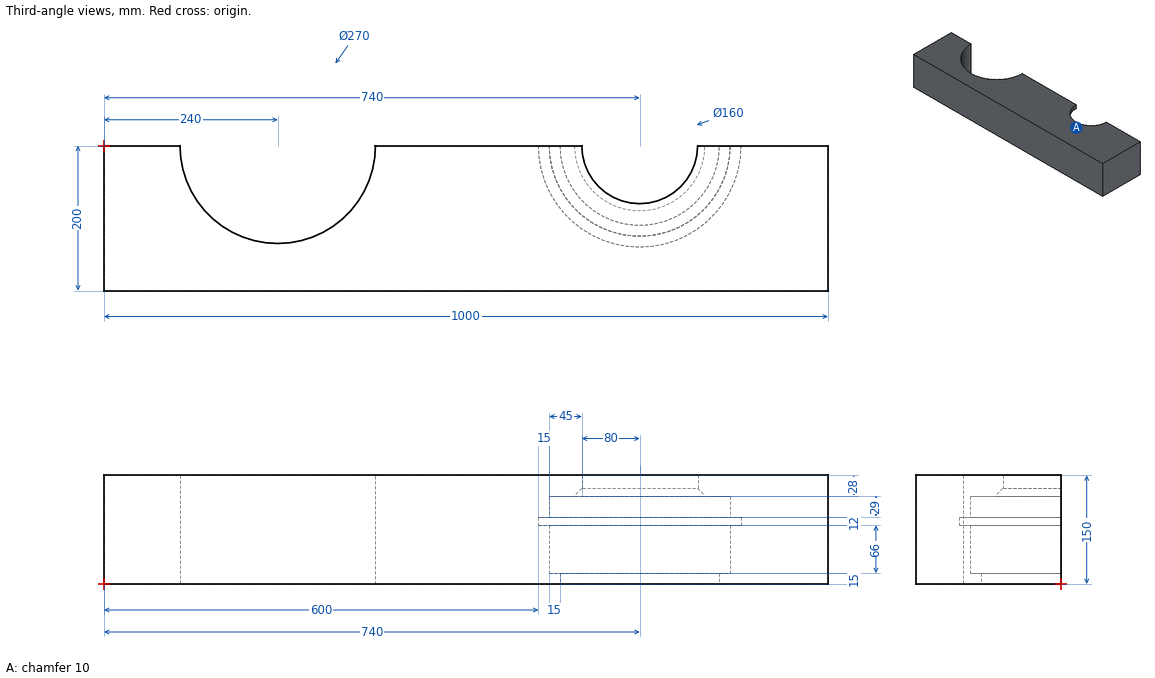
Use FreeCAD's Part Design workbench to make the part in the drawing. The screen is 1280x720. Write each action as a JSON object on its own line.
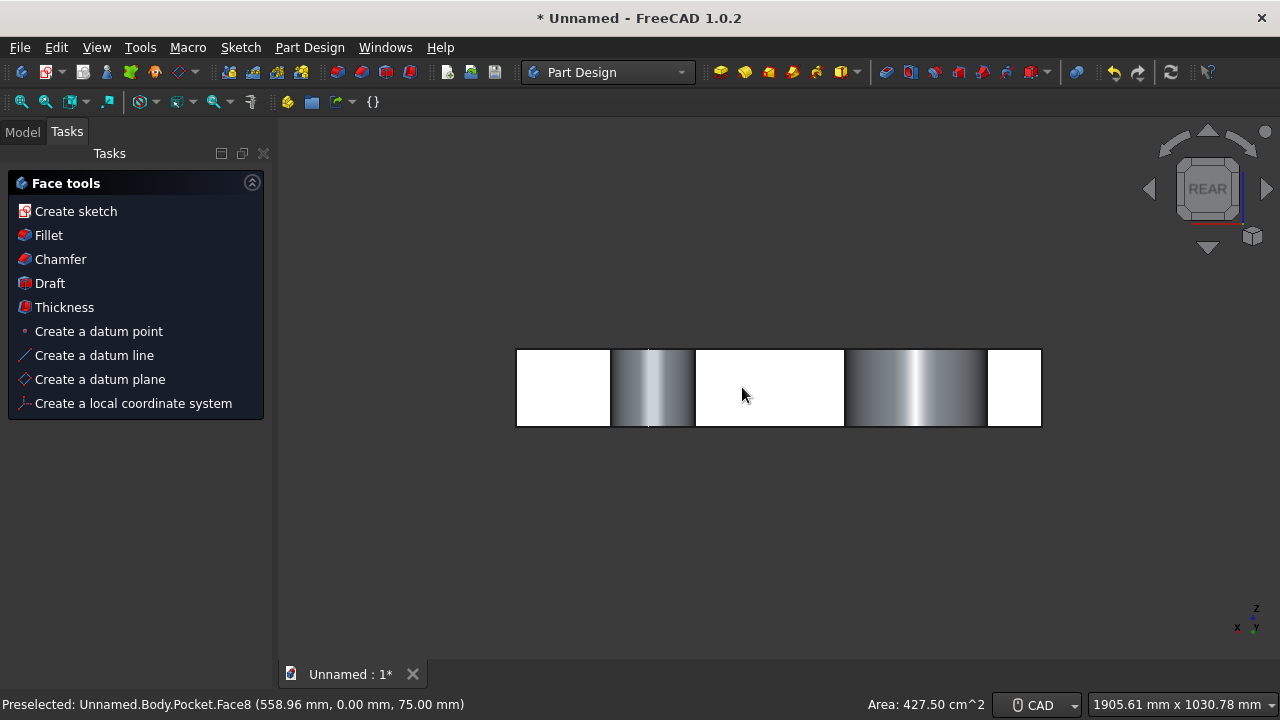
{"action": "left_click", "coordinate": [46, 72]}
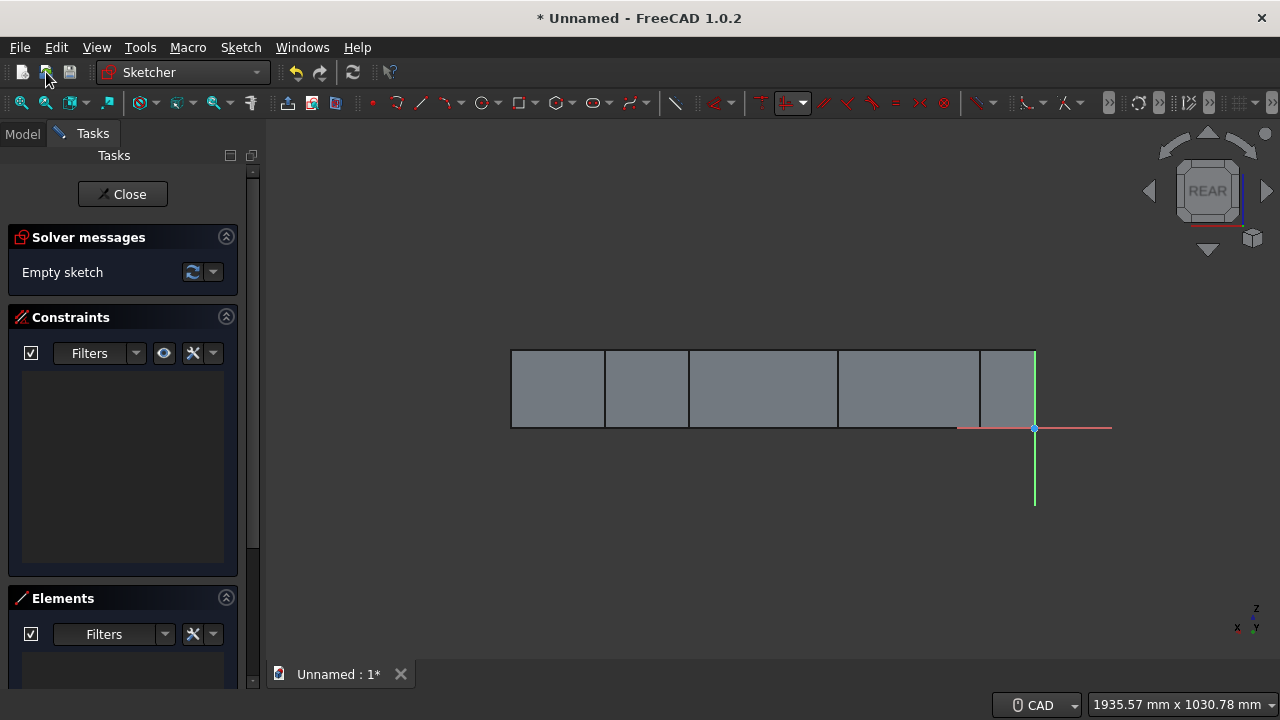
{"action": "scroll", "coordinate": [675, 367], "scroll_direction": "up", "scroll_amount": 6}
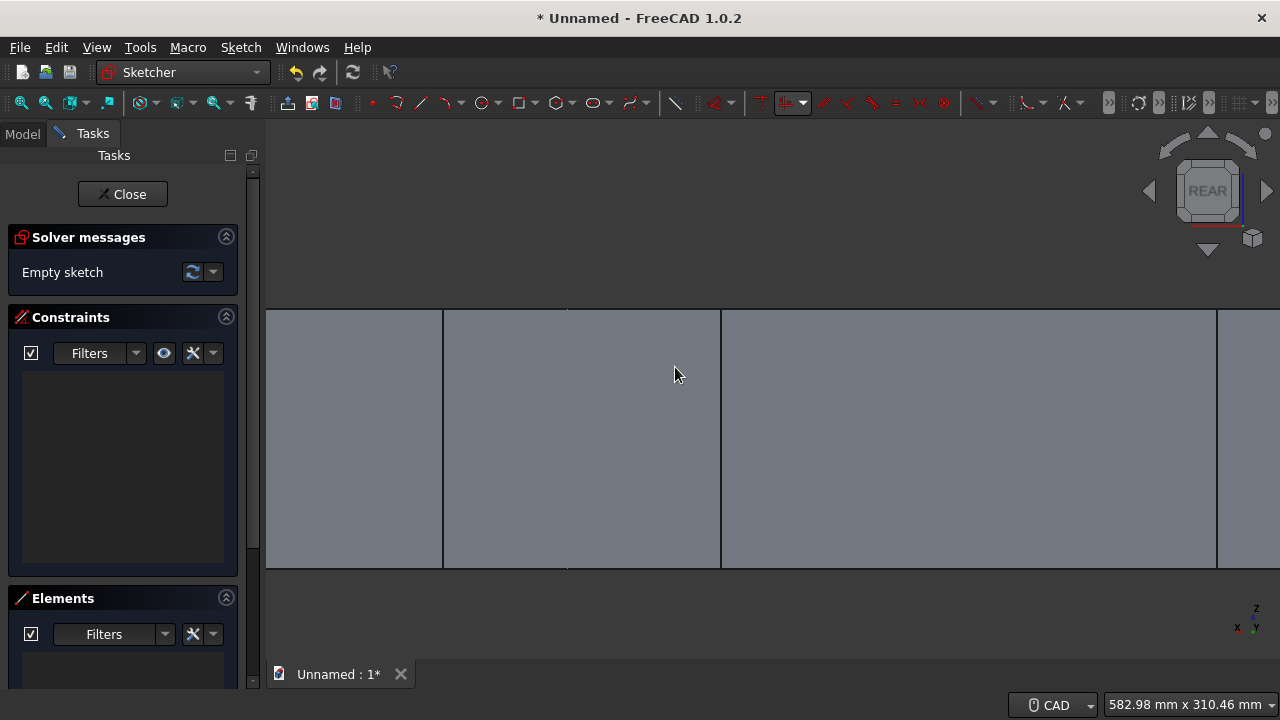
{"action": "left_click", "coordinate": [398, 104]}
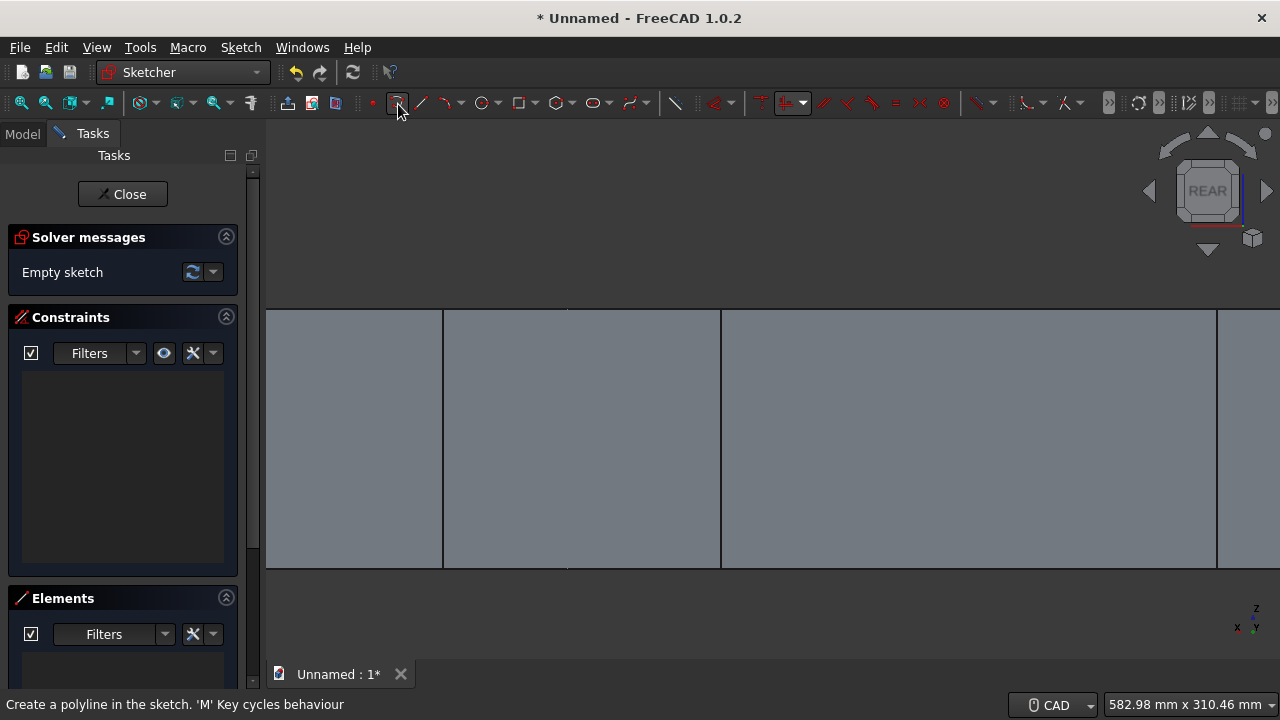
{"action": "left_click", "coordinate": [826, 429]}
{"action": "left_click", "coordinate": [826, 408]}
{"action": "left_click", "coordinate": [799, 408]}
{"action": "left_click", "coordinate": [799, 357]}
{"action": "left_click", "coordinate": [721, 357]}
{"action": "left_click", "coordinate": [721, 309]}
{"action": "left_click", "coordinate": [582, 309]}
{"action": "left_click", "coordinate": [582, 569]}
{"action": "left_click", "coordinate": [773, 560]}
{"action": "left_click", "coordinate": [773, 543]}
{"action": "left_click", "coordinate": [799, 543]}
{"action": "left_click", "coordinate": [799, 429]}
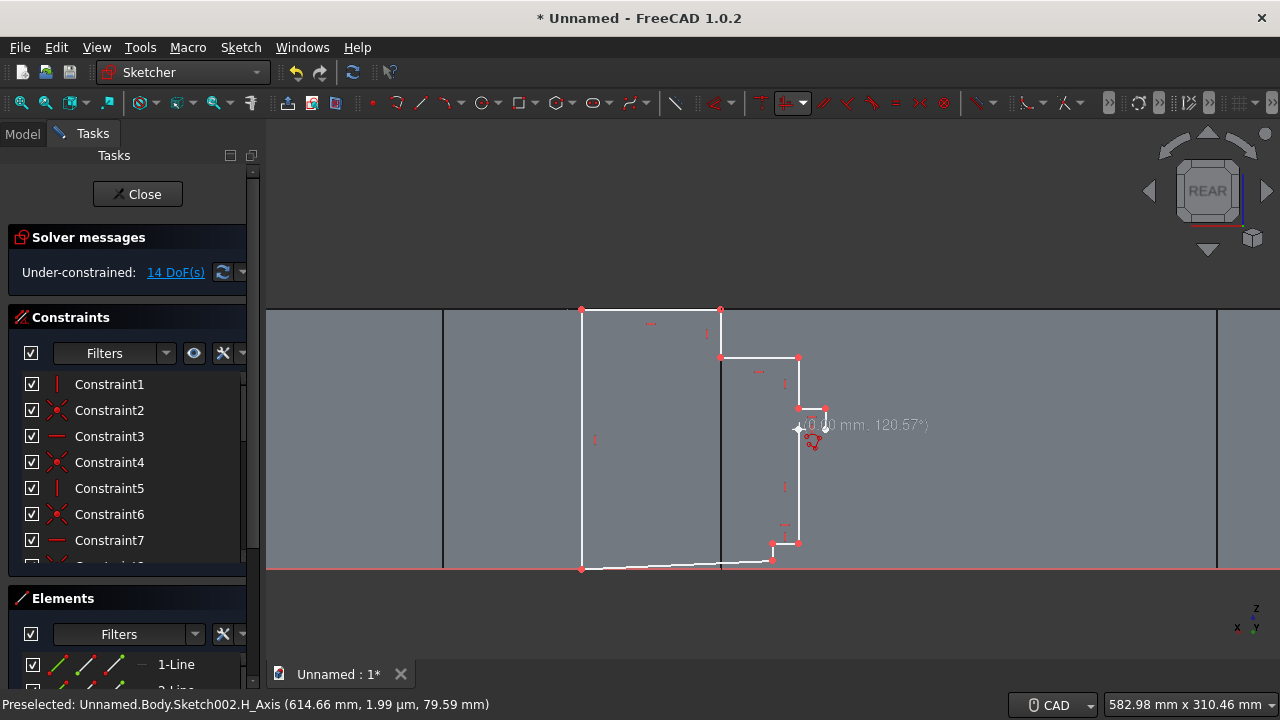
{"action": "scroll", "coordinate": [826, 429], "scroll_direction": "up", "scroll_amount": 3}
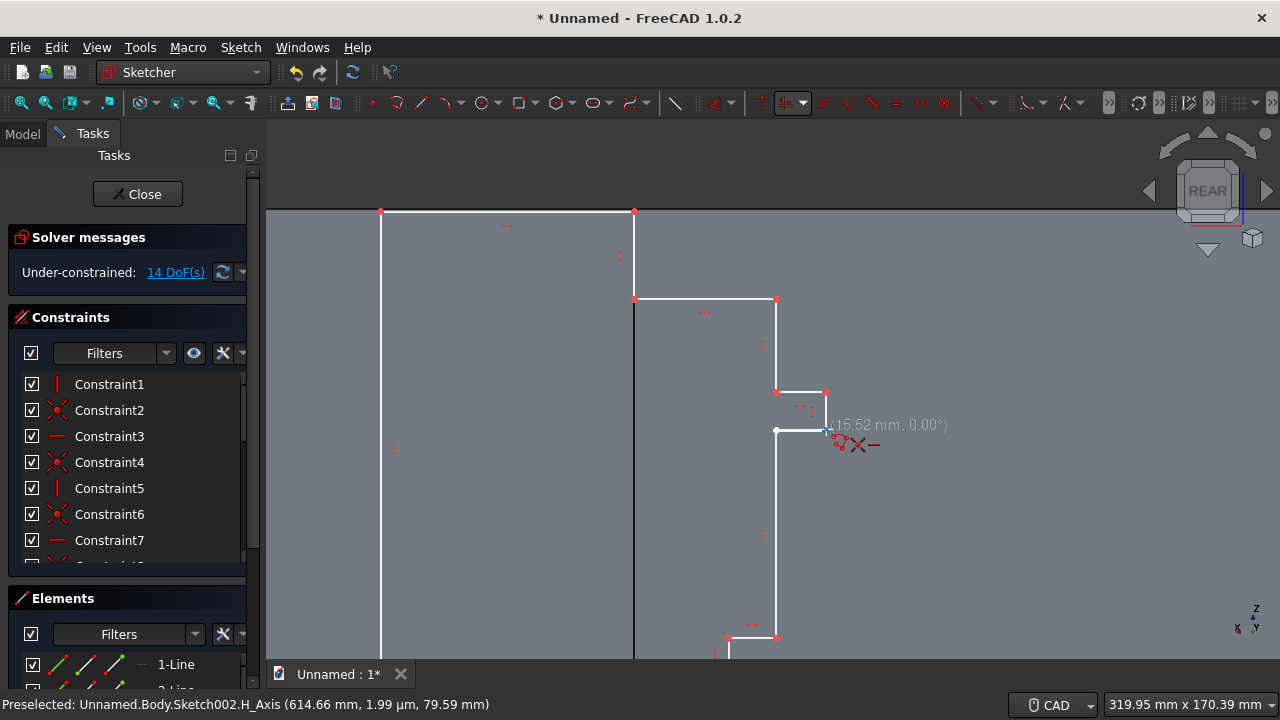
{"action": "left_click", "coordinate": [826, 430]}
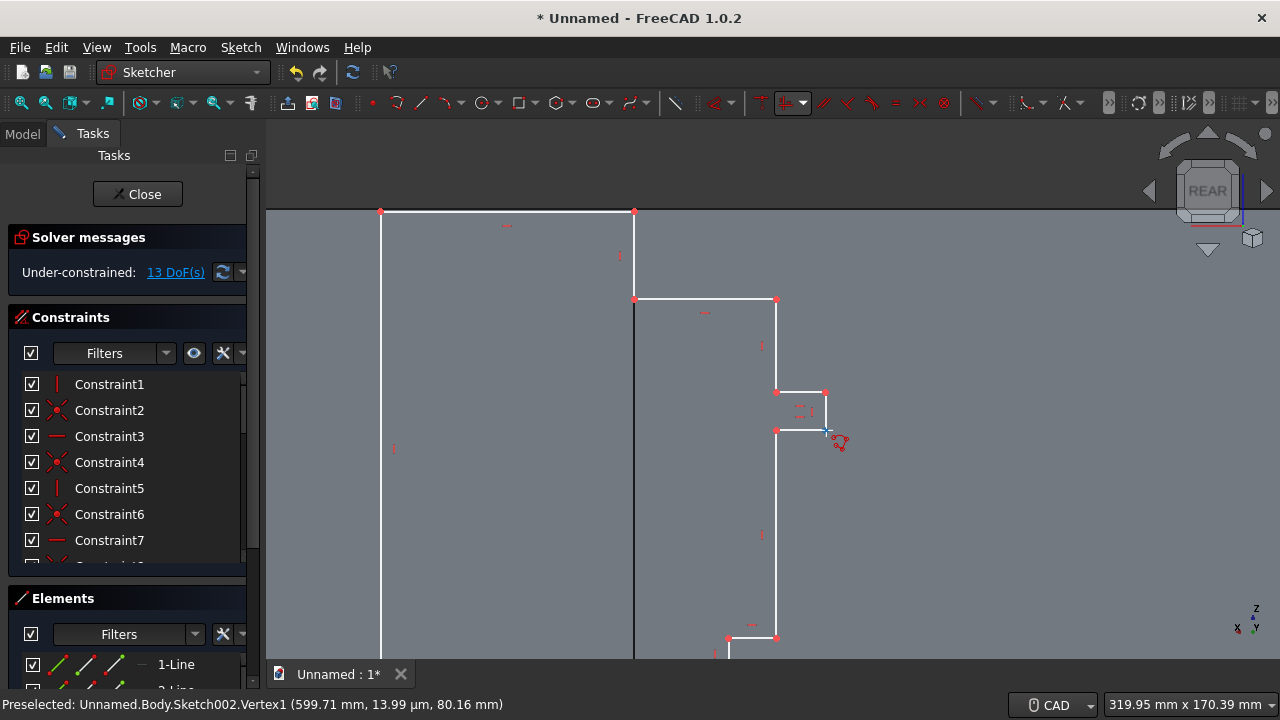
{"action": "left_click", "coordinate": [422, 104]}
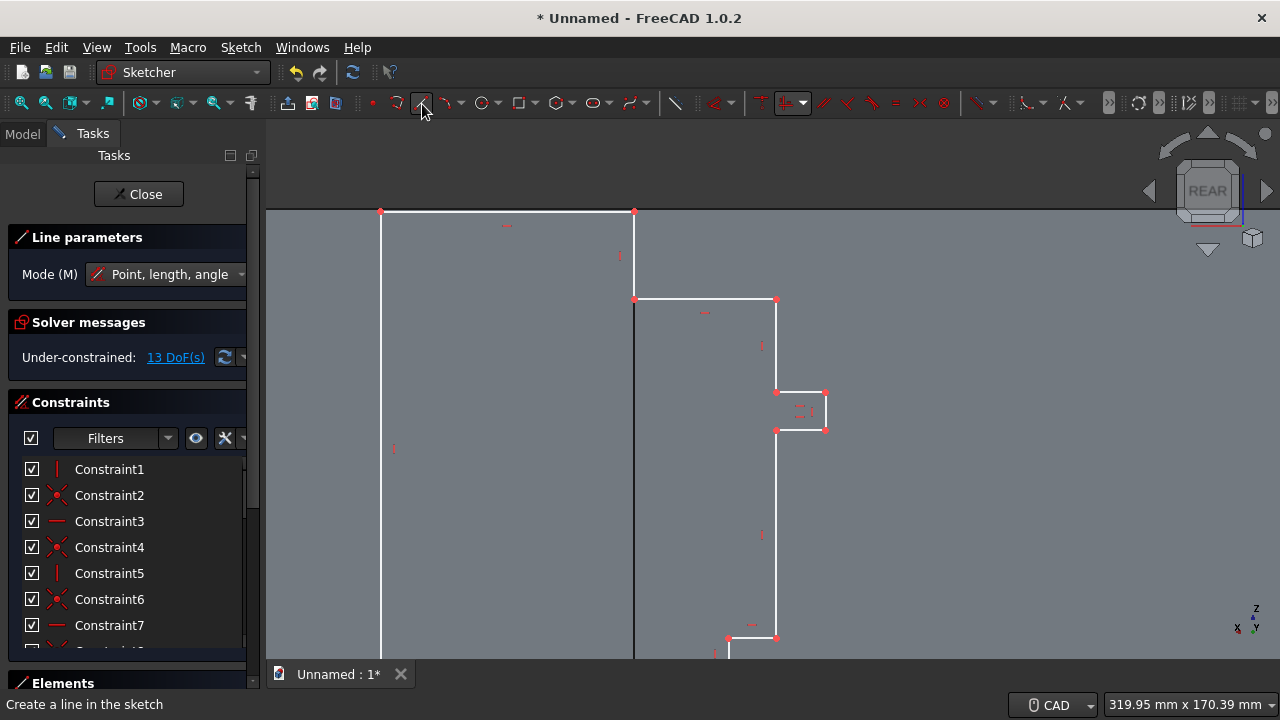
{"action": "left_click", "coordinate": [381, 161]}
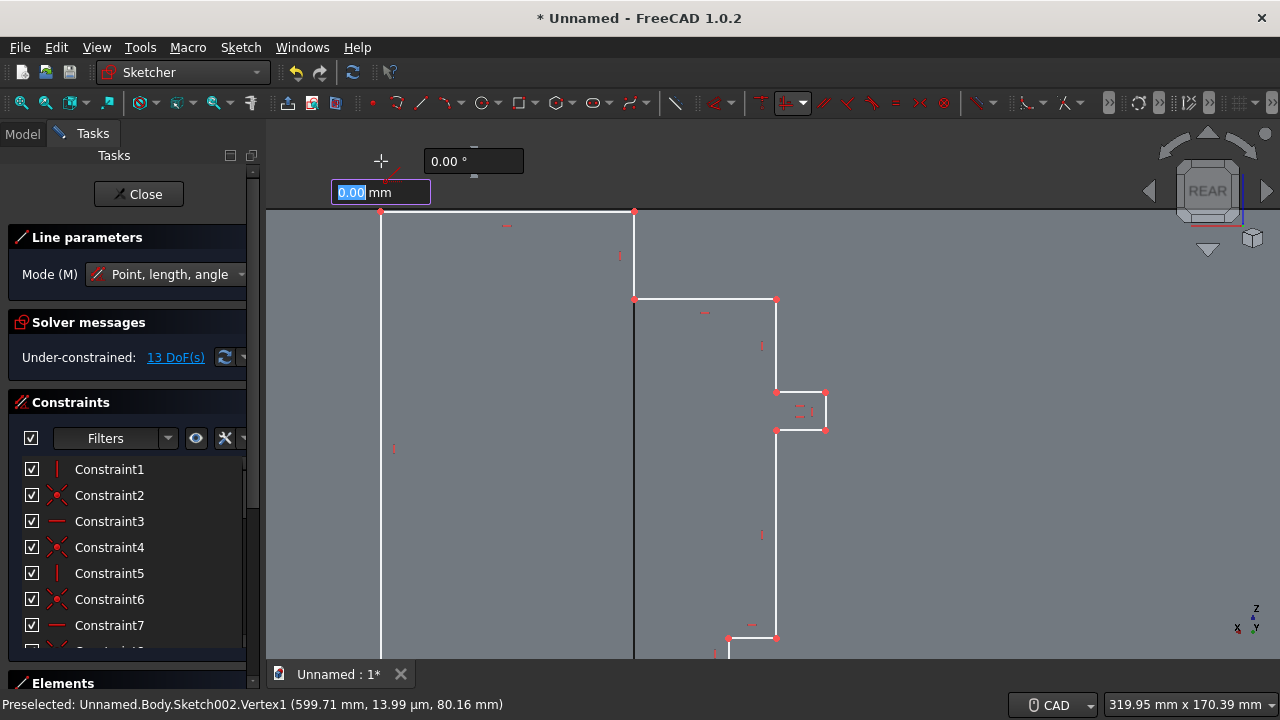
{"action": "scroll", "coordinate": [828, 434], "scroll_direction": "down", "scroll_amount": 3}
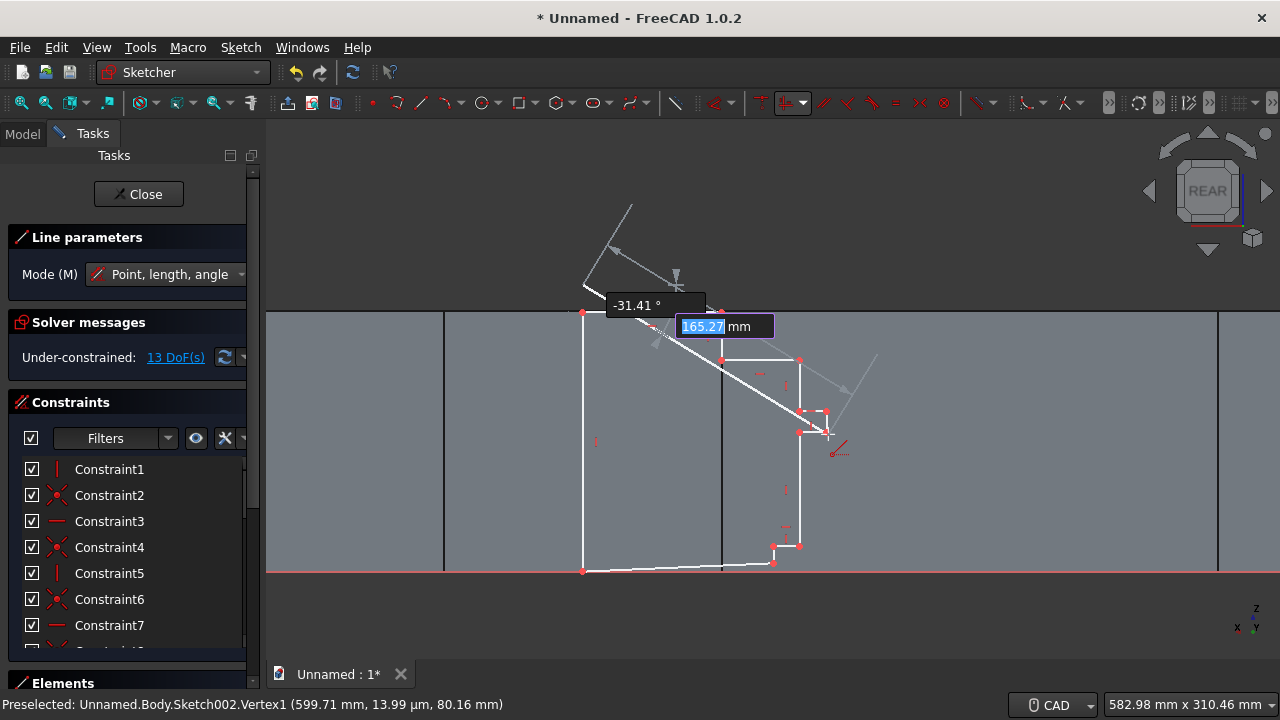
{"action": "left_click", "coordinate": [583, 206]}
{"action": "key", "text": "Escape"}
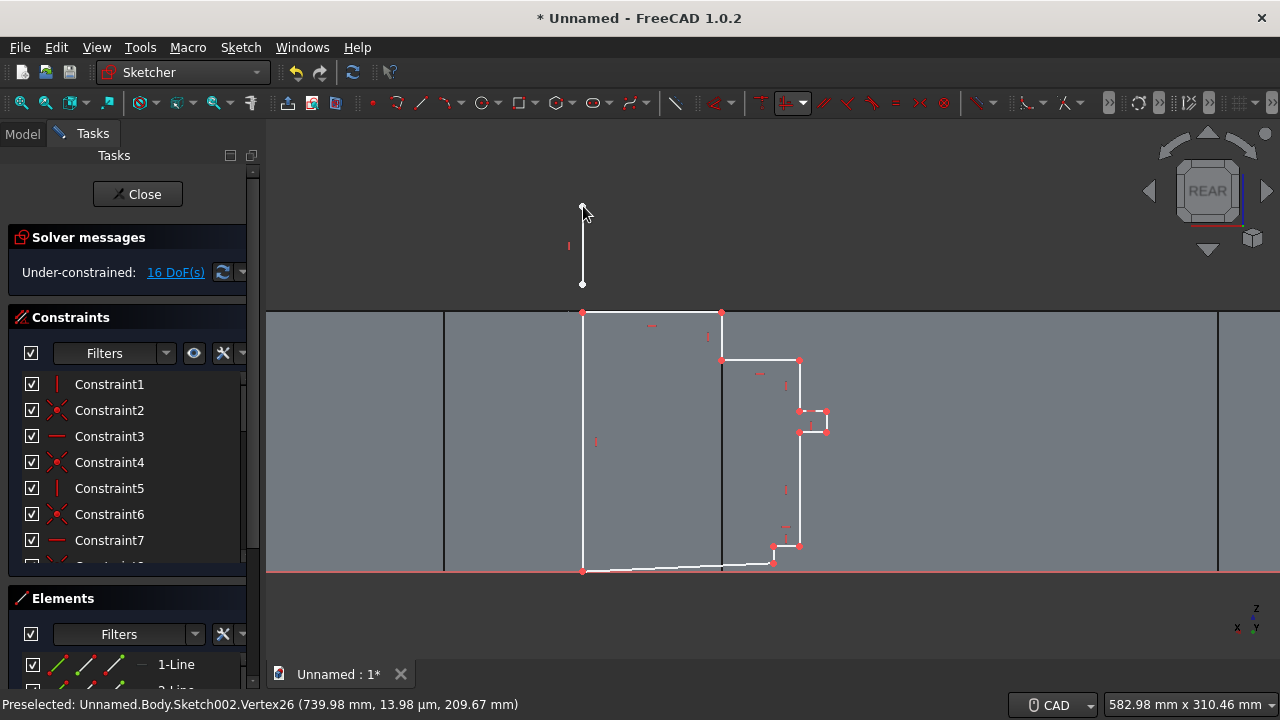
{"action": "left_click", "coordinate": [583, 262]}